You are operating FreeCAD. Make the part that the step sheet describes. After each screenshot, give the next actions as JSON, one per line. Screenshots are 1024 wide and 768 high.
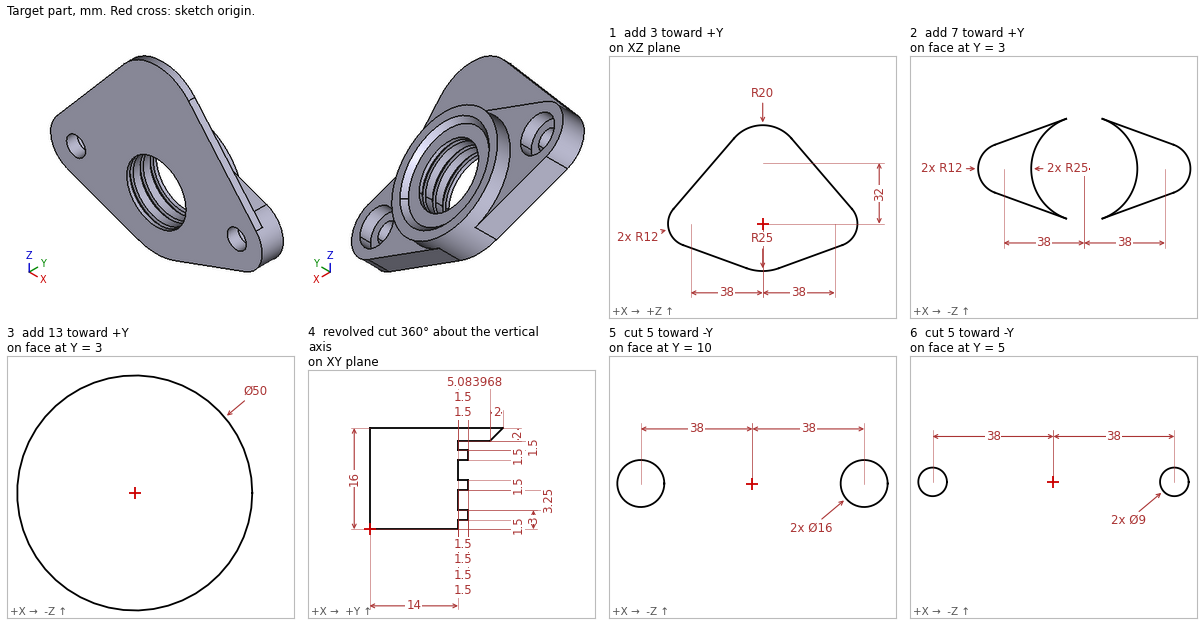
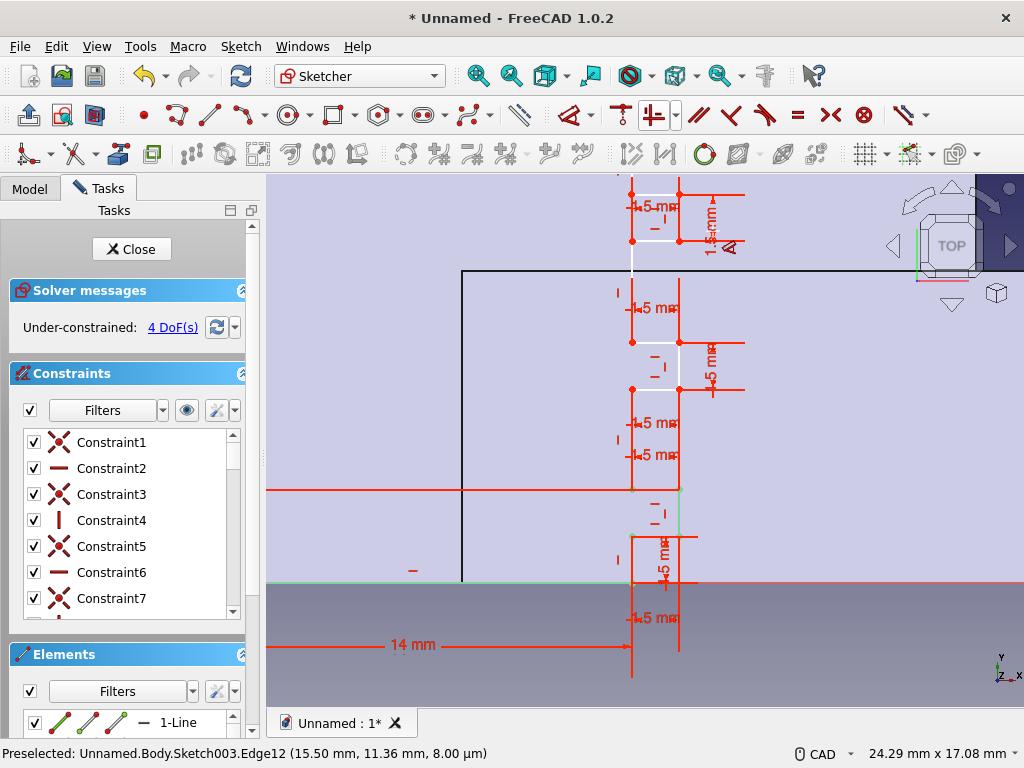
{"action": "scroll", "coordinate": [640, 570], "scroll_direction": "down", "scroll_amount": 3}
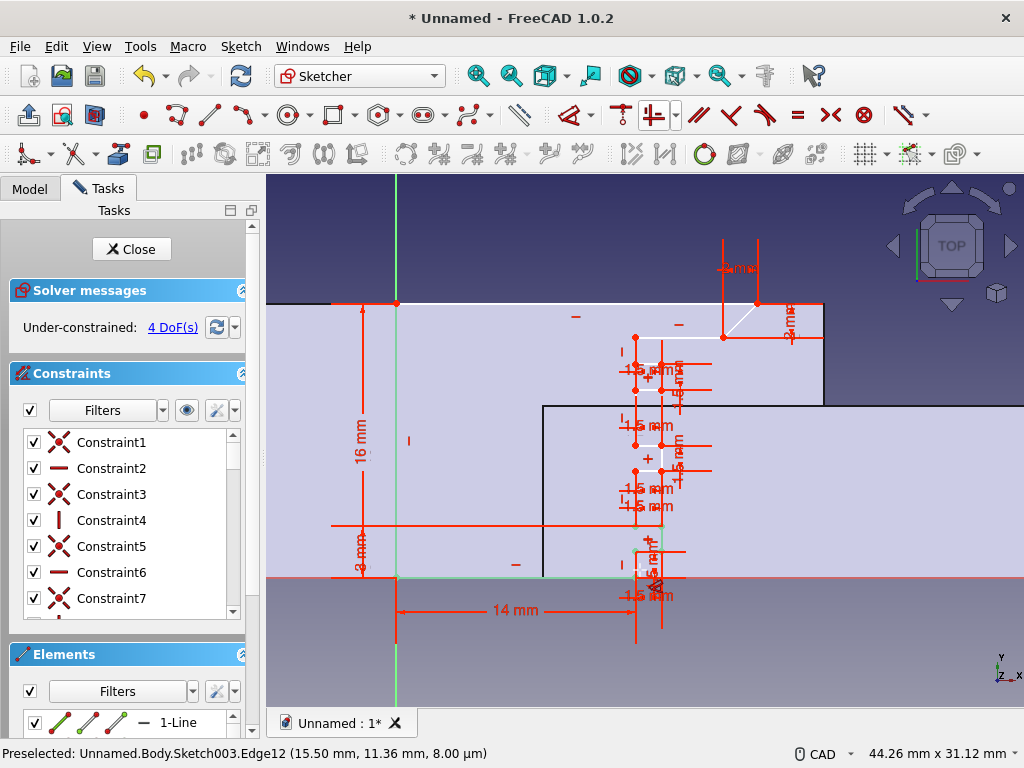
{"action": "scroll", "coordinate": [654, 364], "scroll_direction": "up", "scroll_amount": 3}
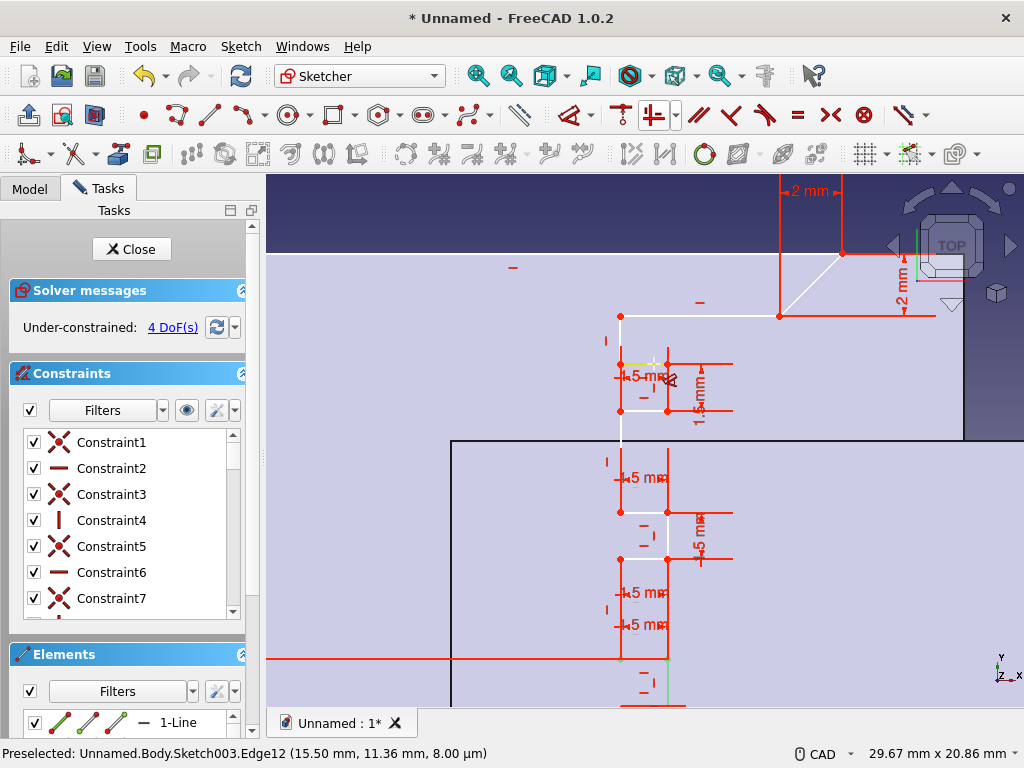
{"action": "left_click", "coordinate": [653, 364]}
{"action": "left_click", "coordinate": [644, 330]}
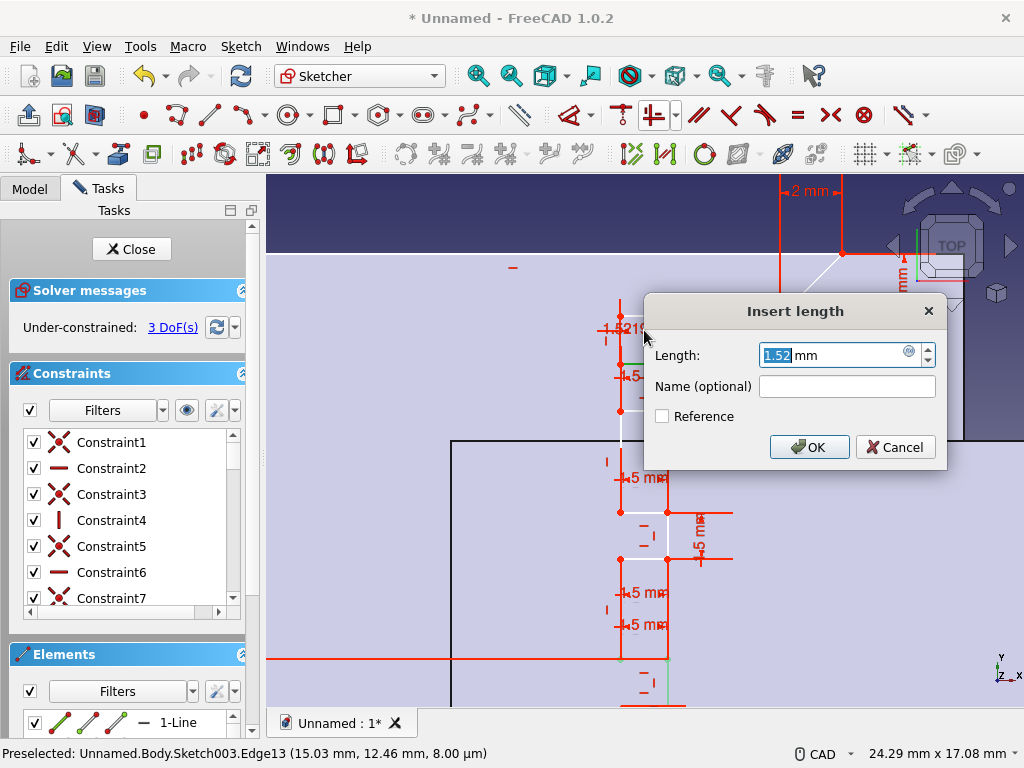
{"action": "type", "text": "1.5"}
{"action": "key", "text": "Return"}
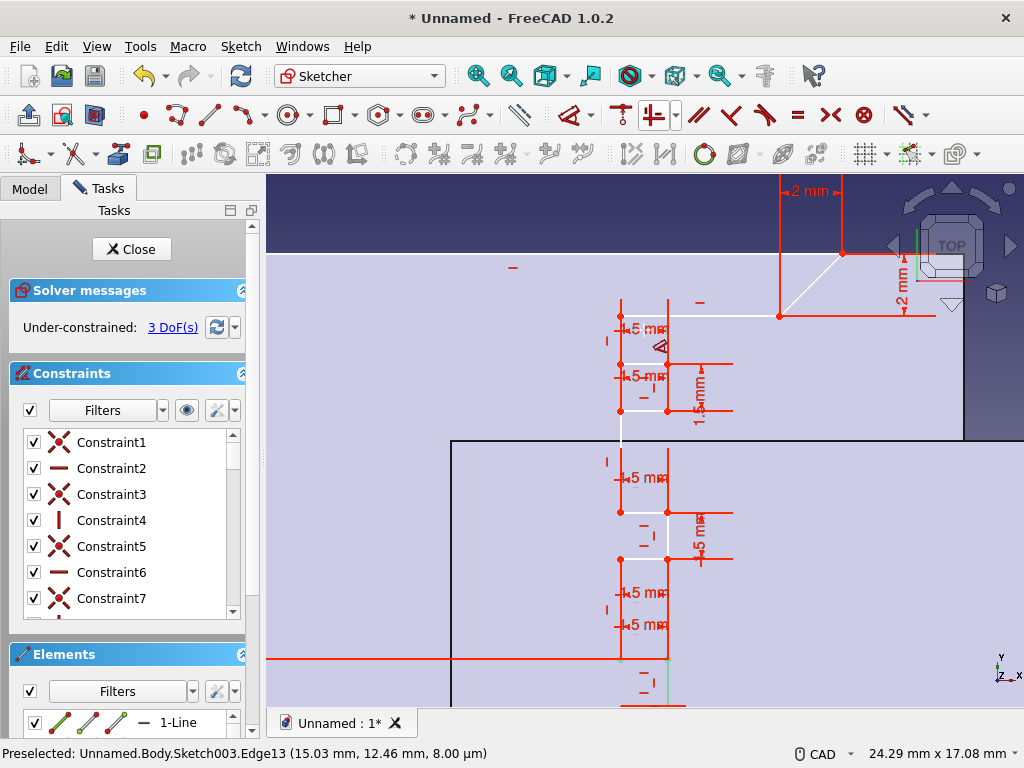
{"action": "left_click", "coordinate": [621, 350]}
{"action": "left_click", "coordinate": [655, 351]}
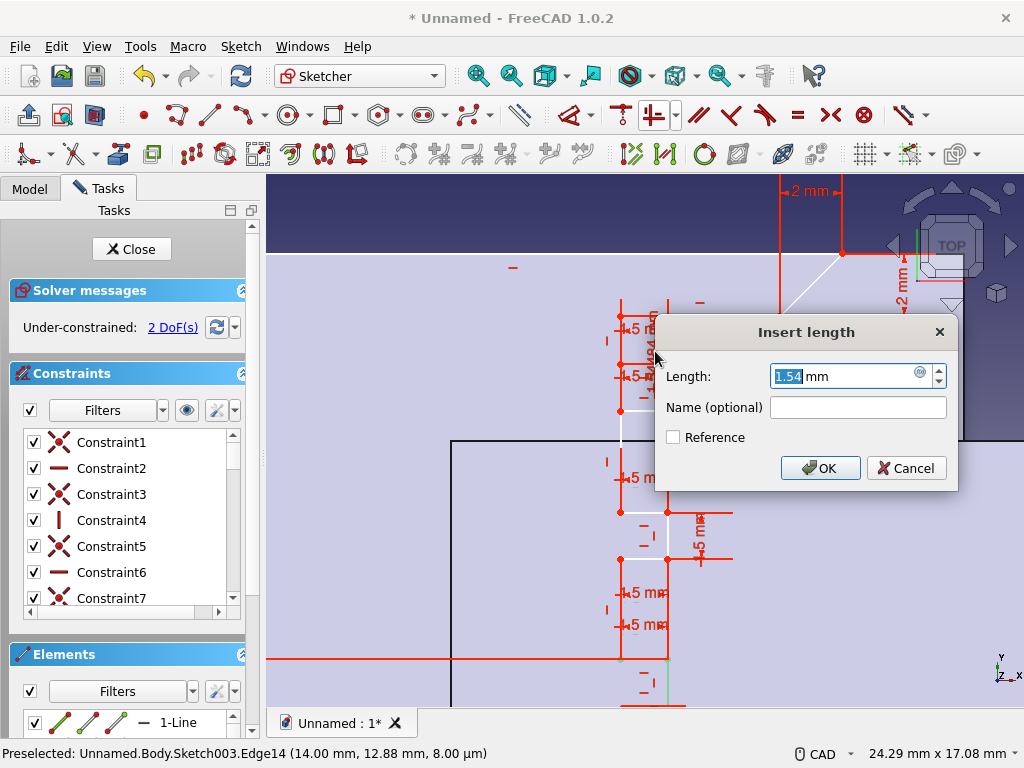
{"action": "type", "text": "1.5"}
{"action": "key", "text": "Return"}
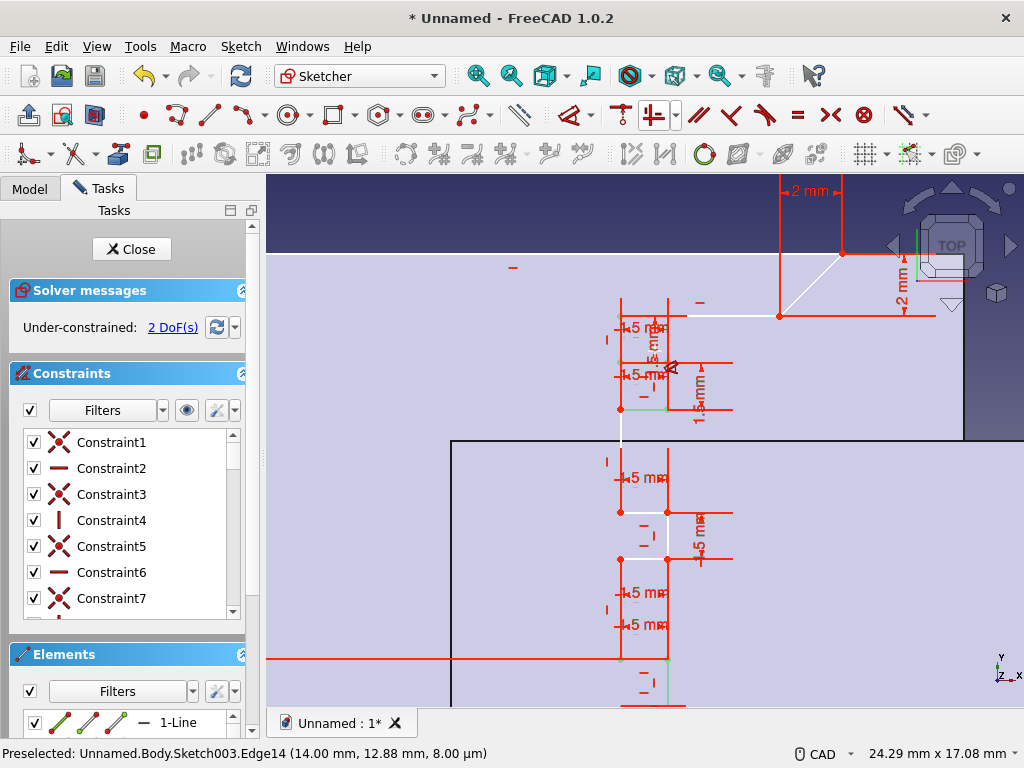
{"action": "left_click", "coordinate": [621, 629]}
{"action": "left_click", "coordinate": [563, 609]}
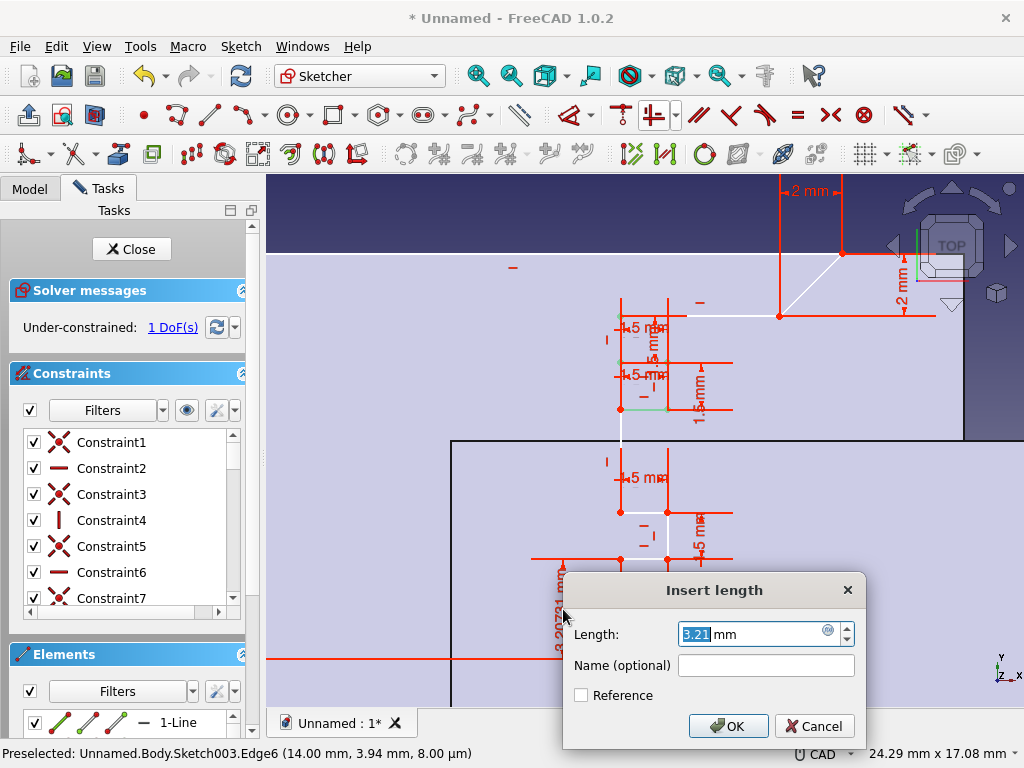
{"action": "type", "text": "3.25"}
{"action": "key", "text": "Return"}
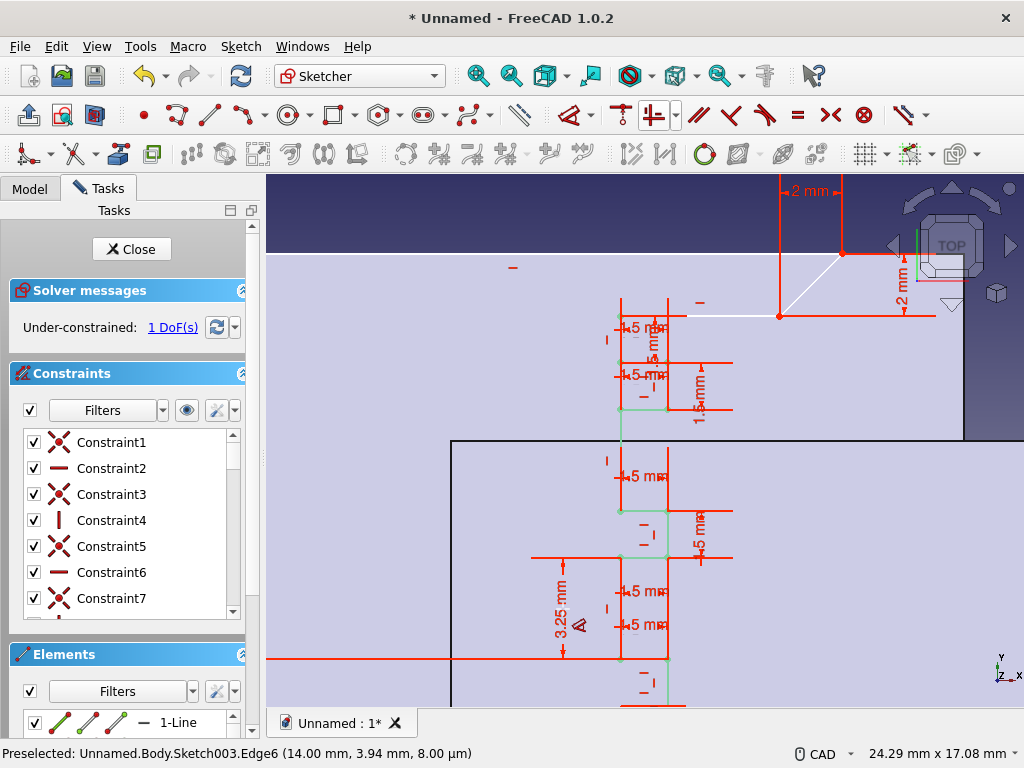
{"action": "left_click", "coordinate": [669, 316]}
{"action": "left_click", "coordinate": [700, 282]}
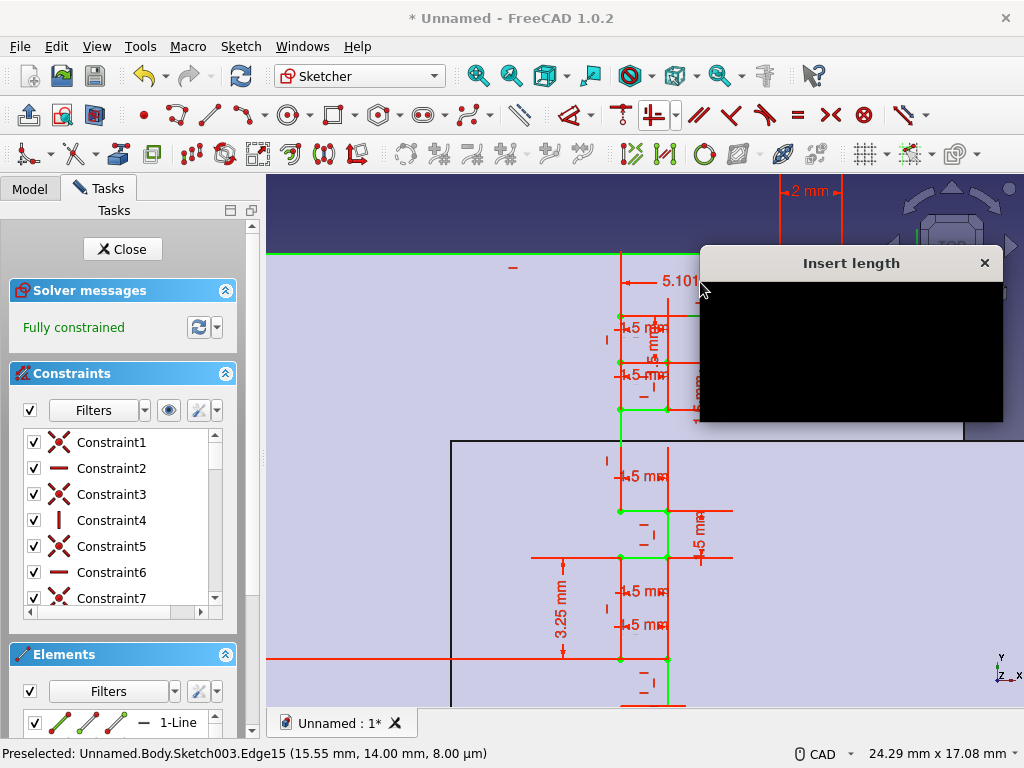
{"action": "type", "text": "5.083968"}
{"action": "key", "text": "Return"}
{"action": "key", "text": "Escape"}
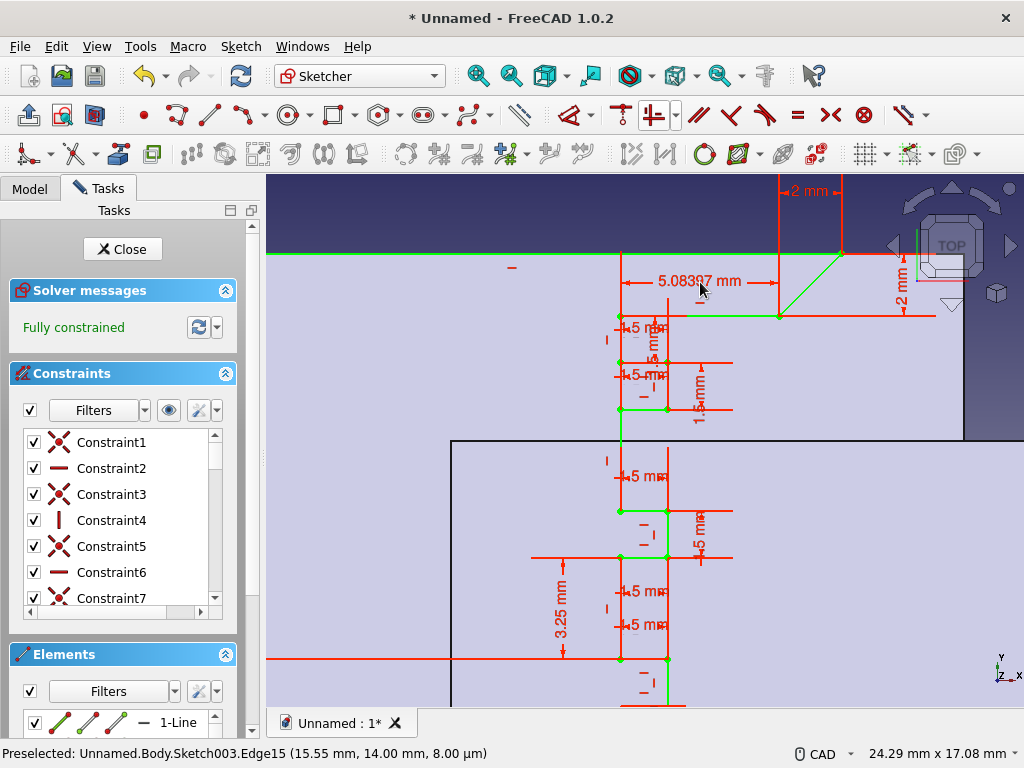
{"action": "left_click", "coordinate": [123, 249]}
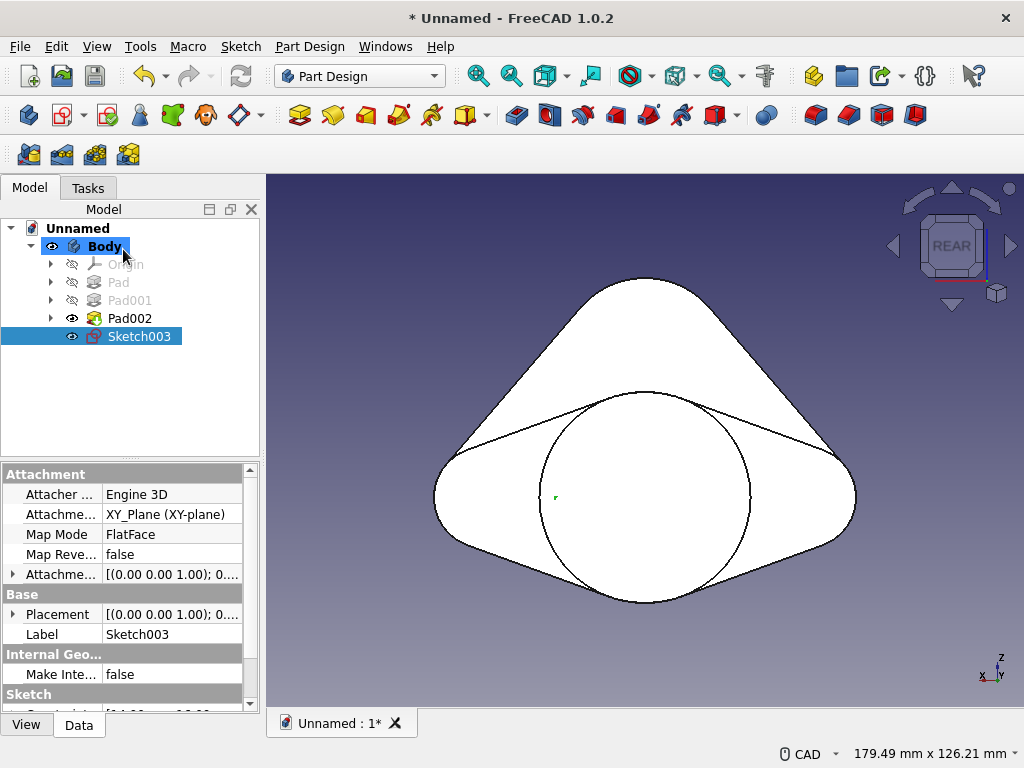
{"action": "left_click", "coordinate": [583, 116]}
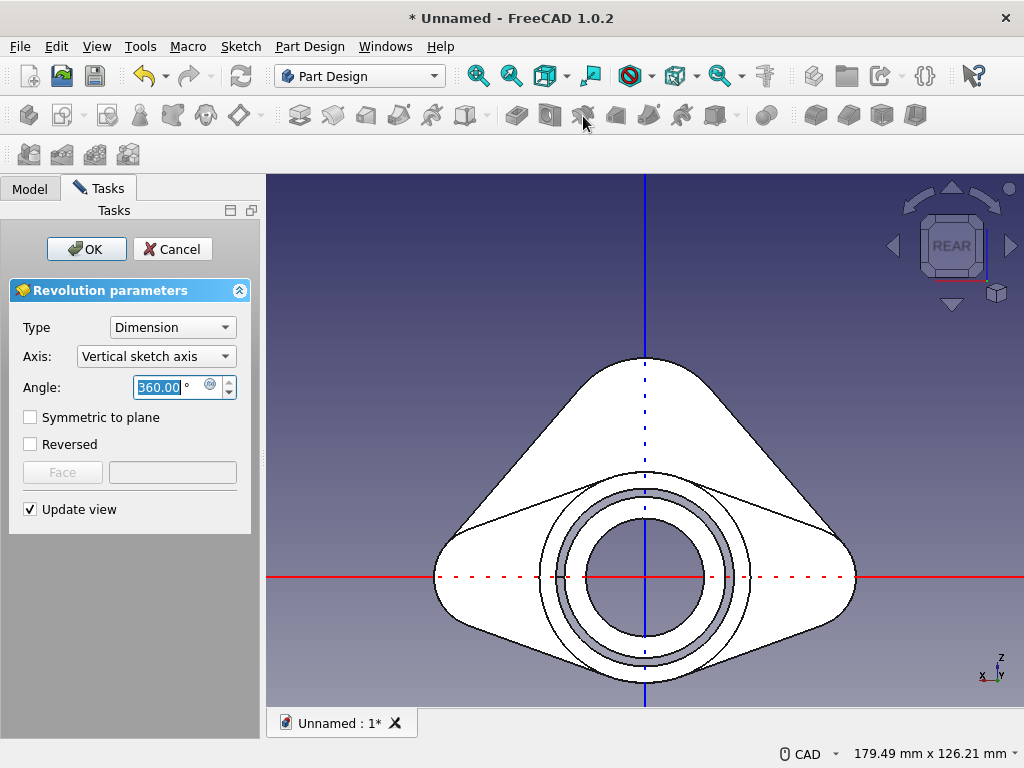
{"action": "left_click", "coordinate": [87, 249]}